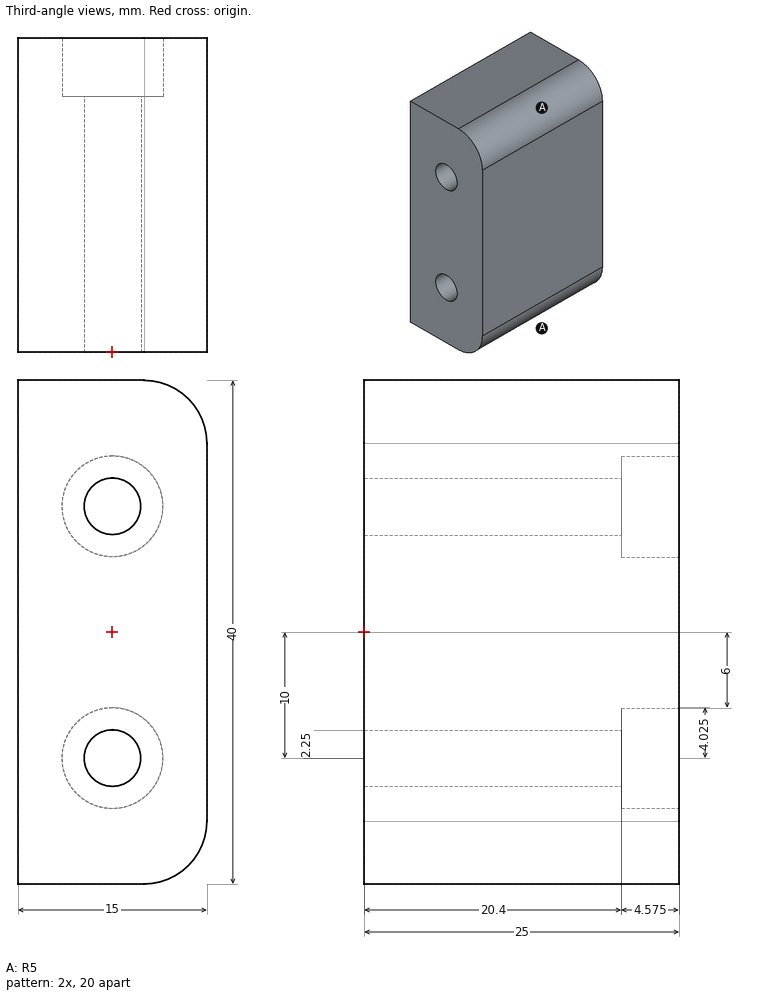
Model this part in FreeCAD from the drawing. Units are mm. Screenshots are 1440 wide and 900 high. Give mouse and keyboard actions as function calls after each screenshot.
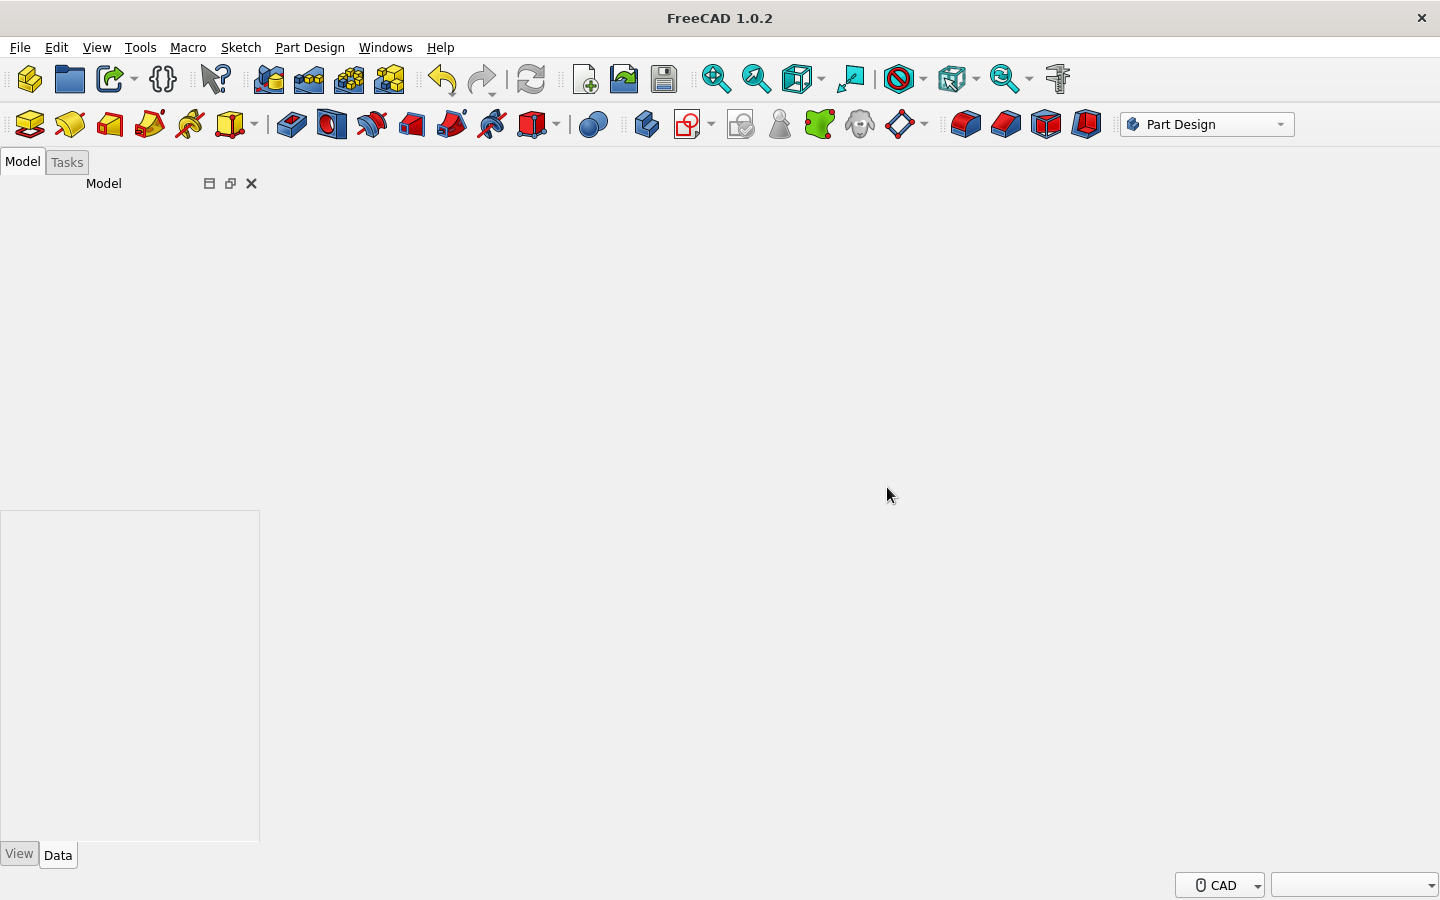
key(ctrl+n)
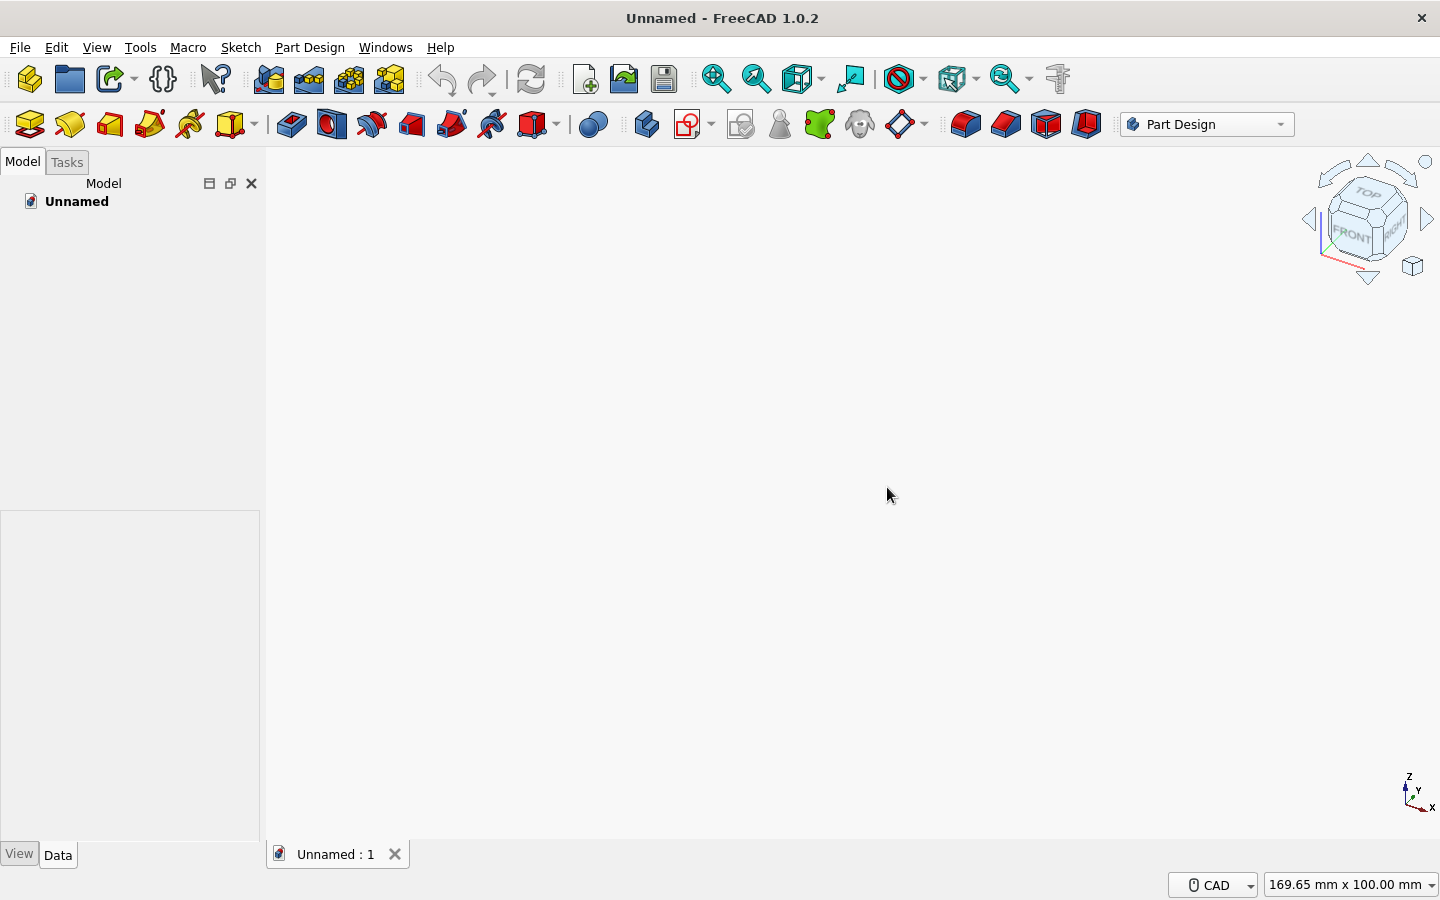
click(688, 124)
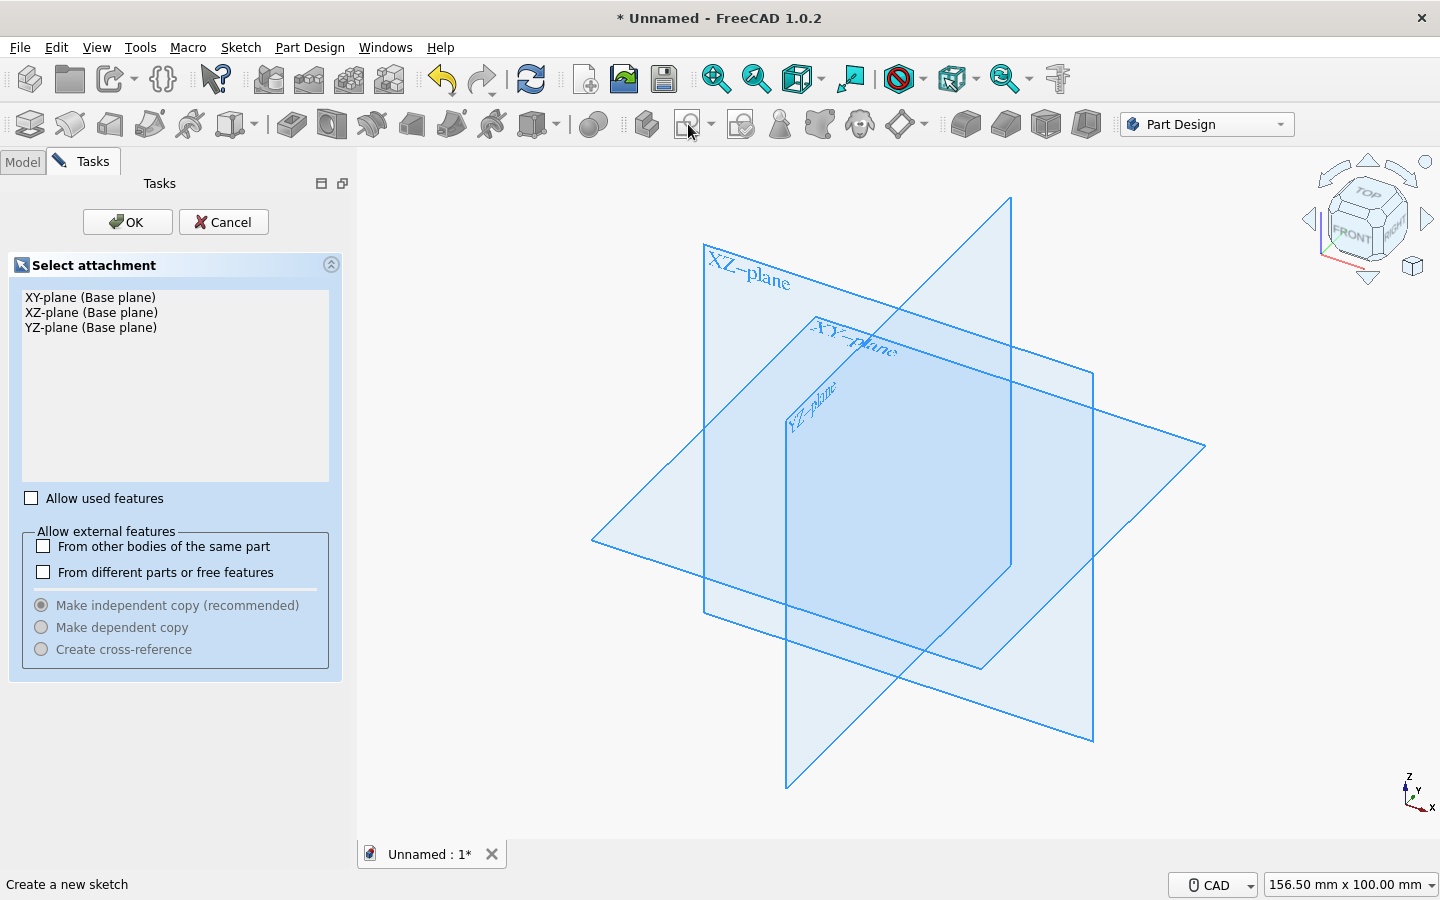
click(82, 312)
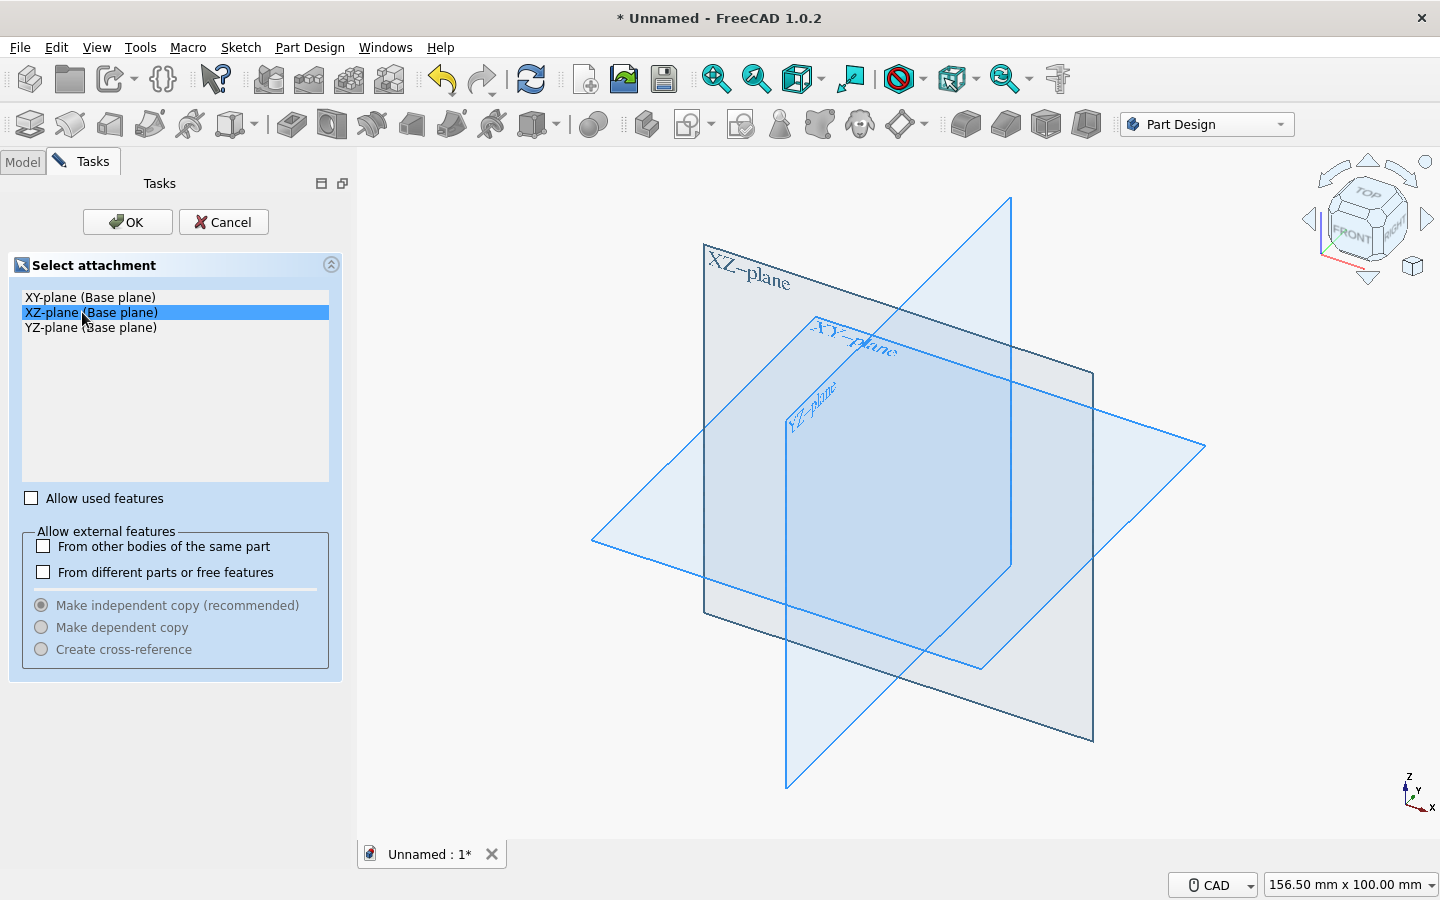
click(128, 222)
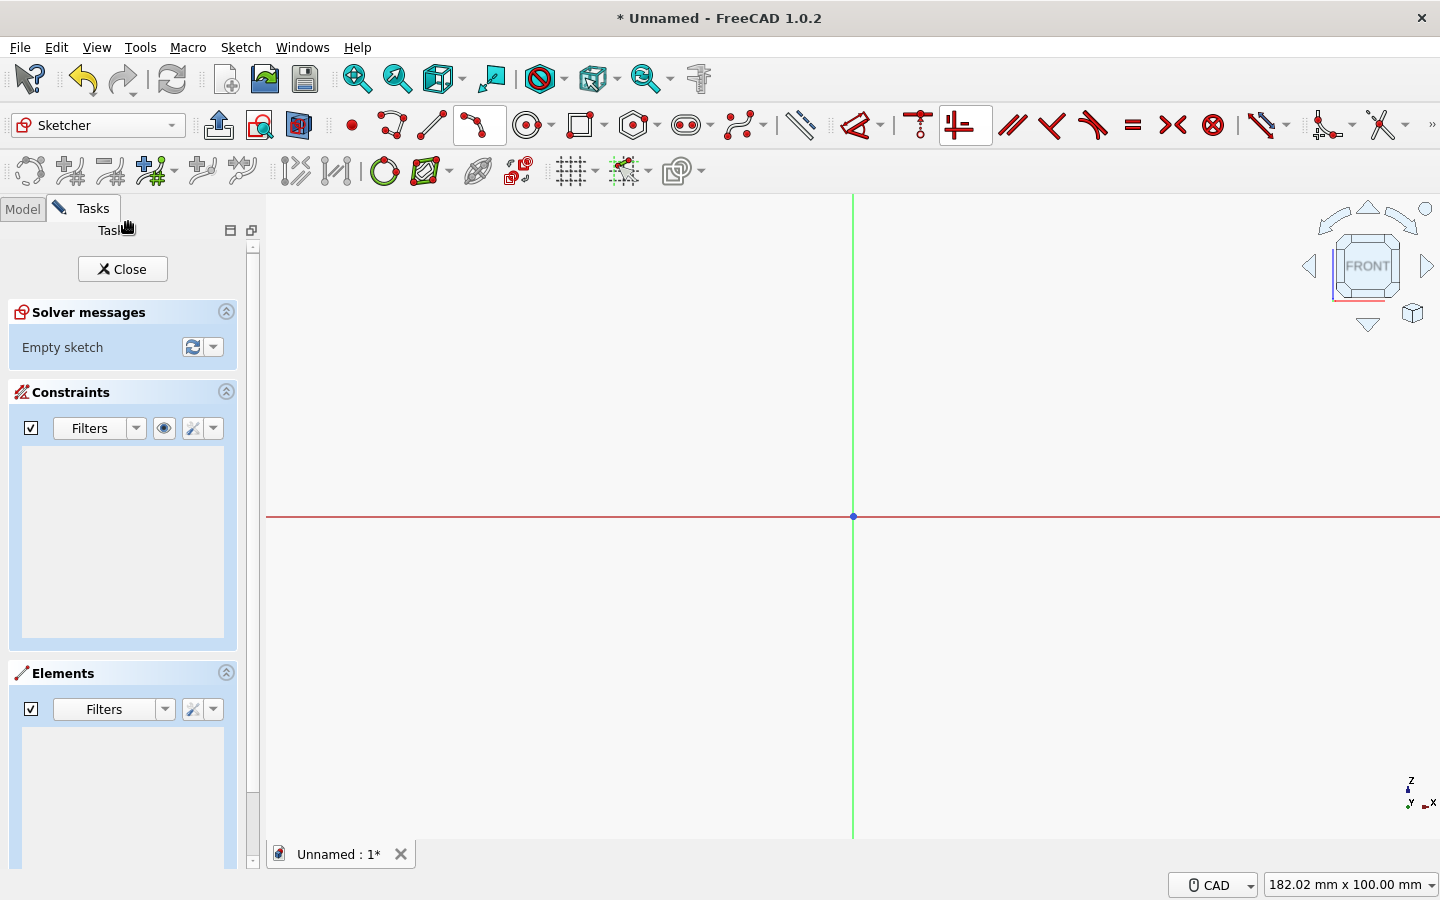
scroll(992, 517, up, 2)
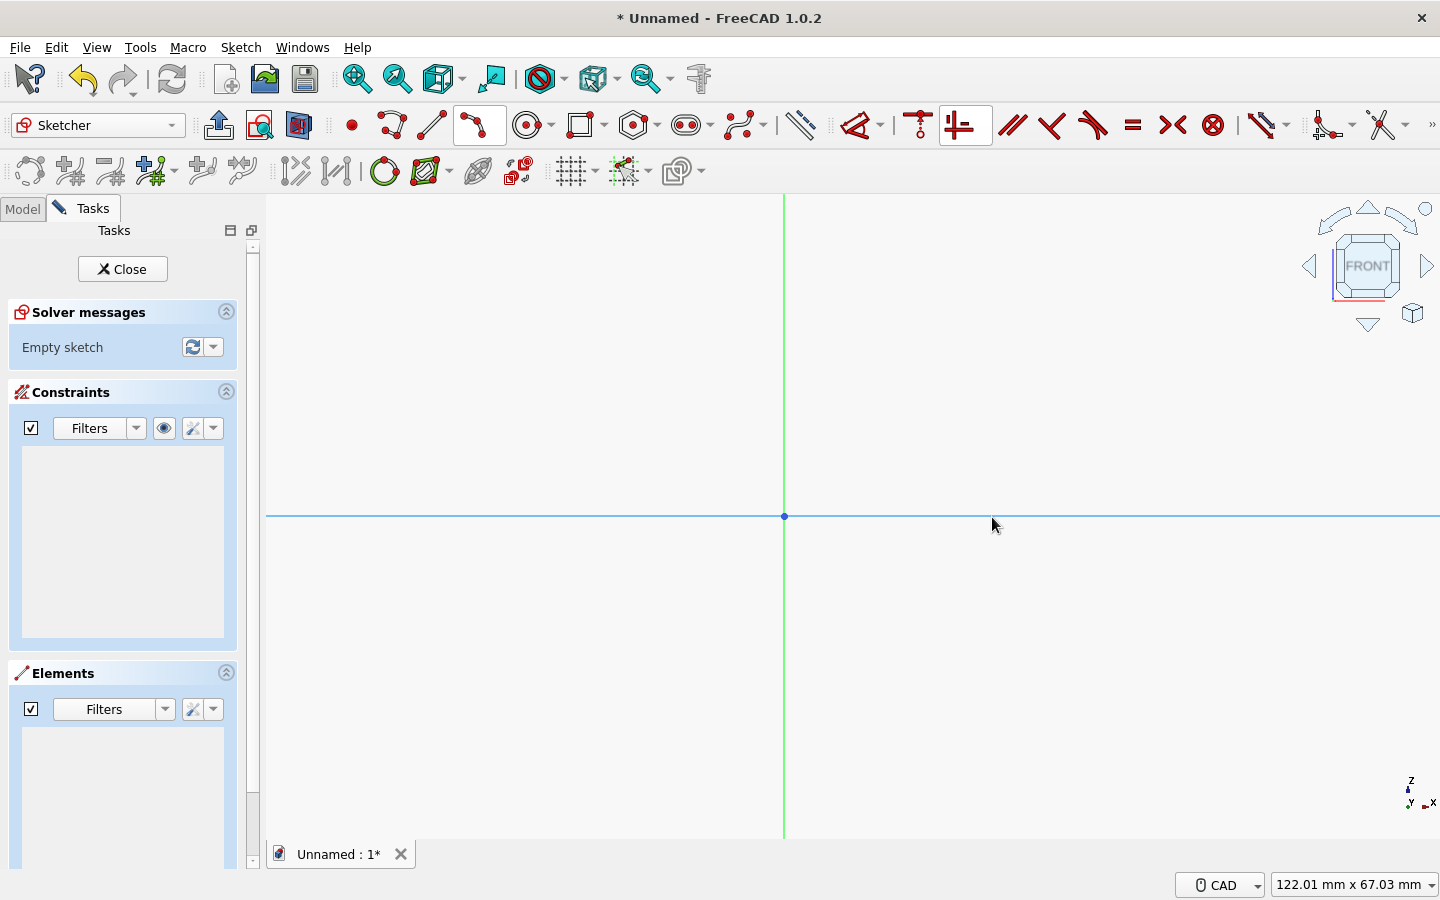
key(g)
key(v)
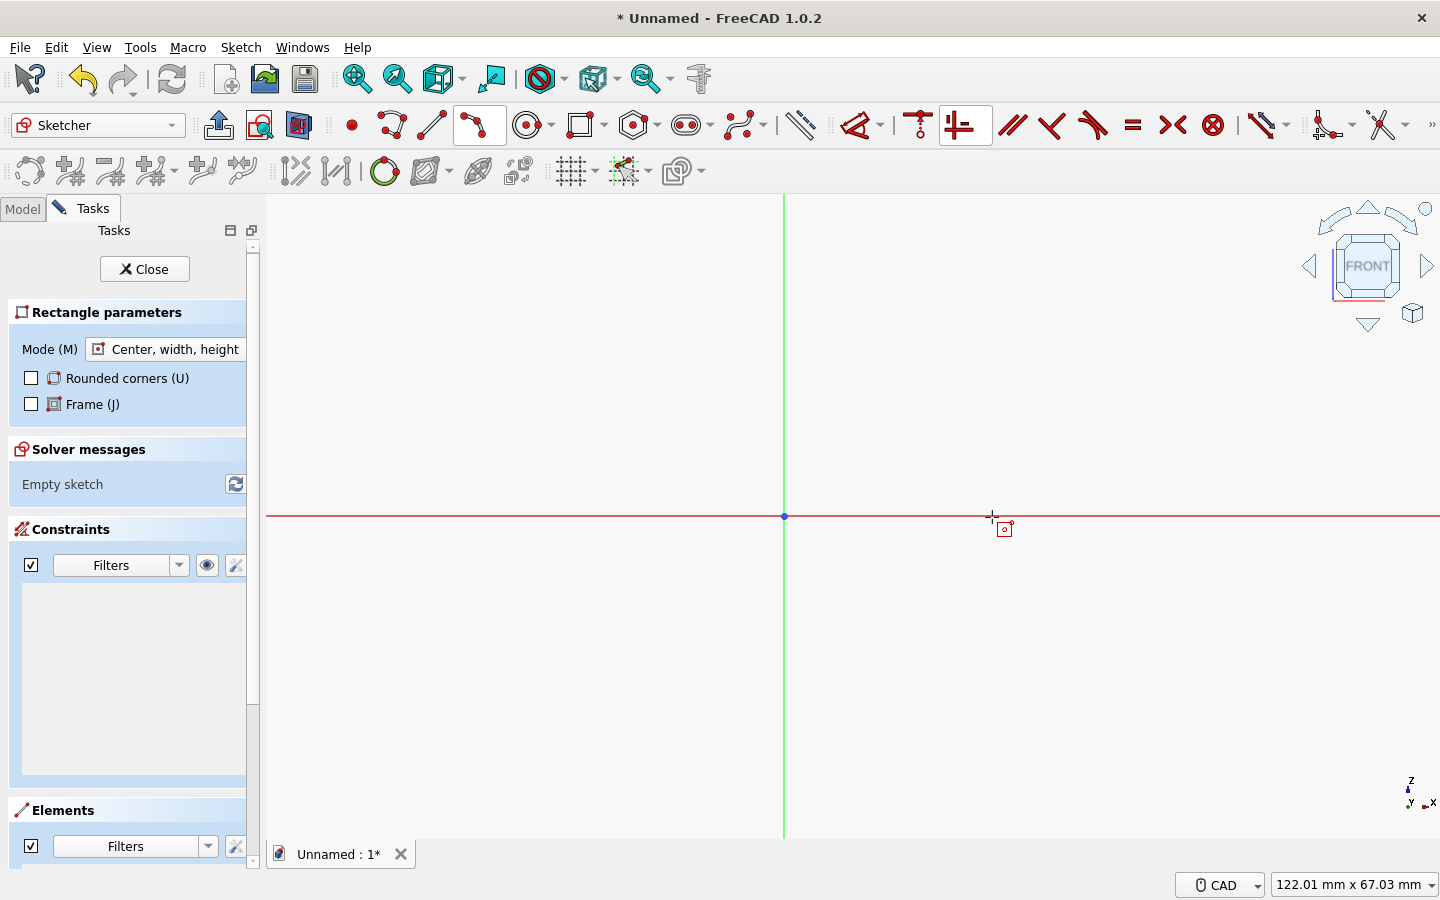
click(784, 516)
move(856, 324)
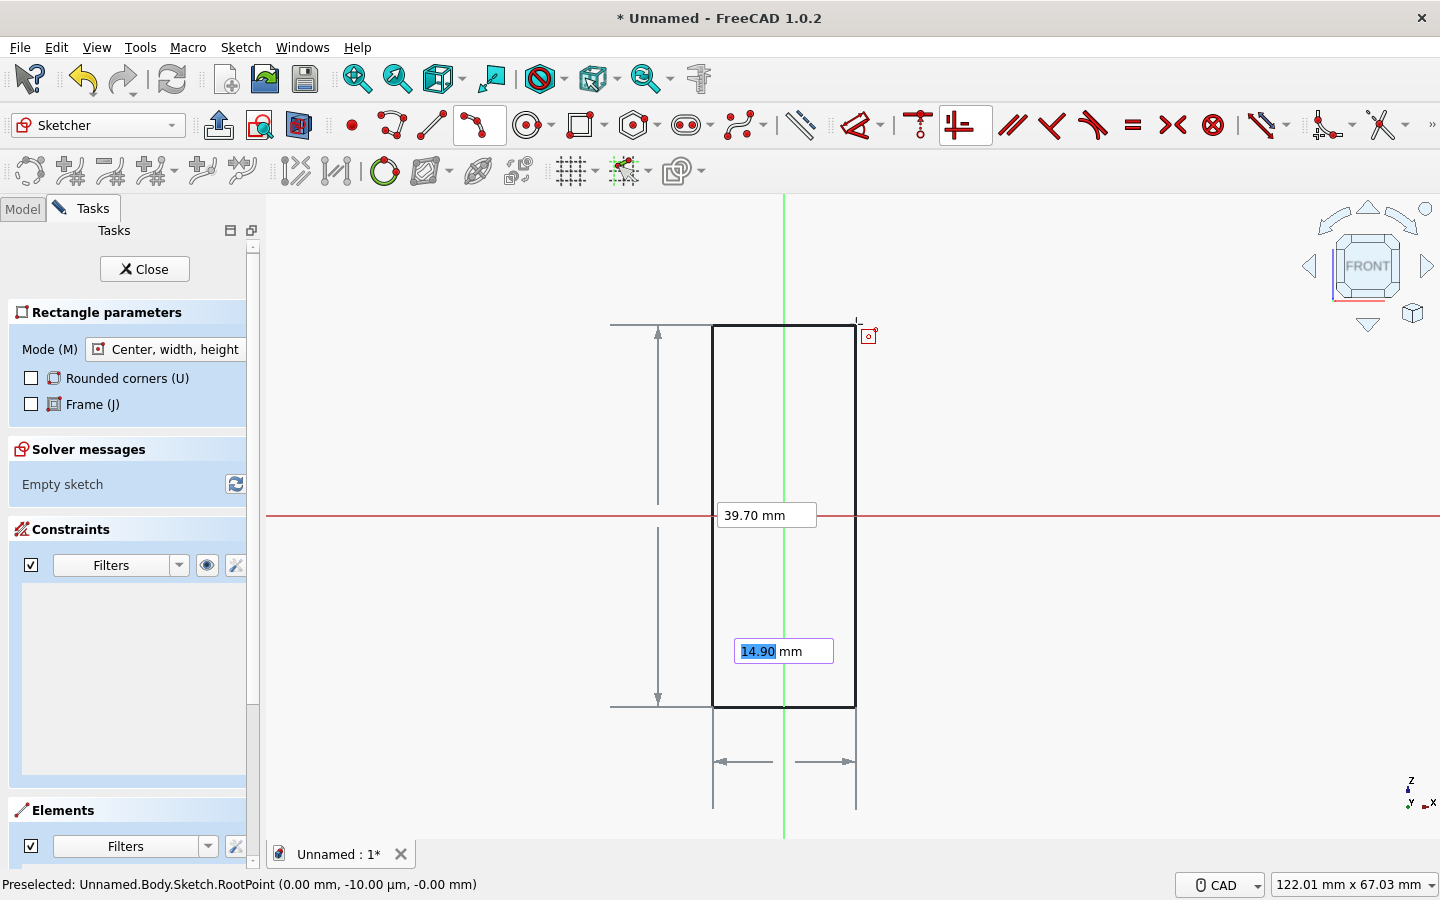
text(15)
key(Tab)
text(40)
key(Return)
key(Escape)